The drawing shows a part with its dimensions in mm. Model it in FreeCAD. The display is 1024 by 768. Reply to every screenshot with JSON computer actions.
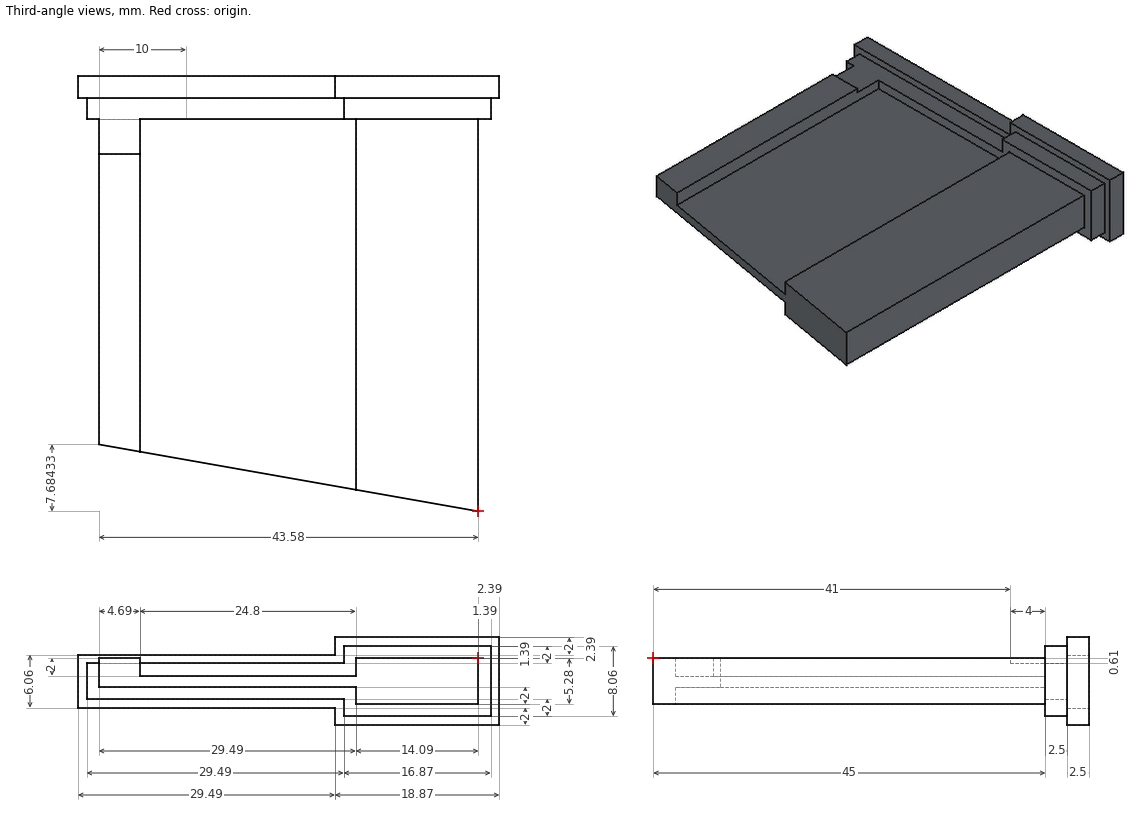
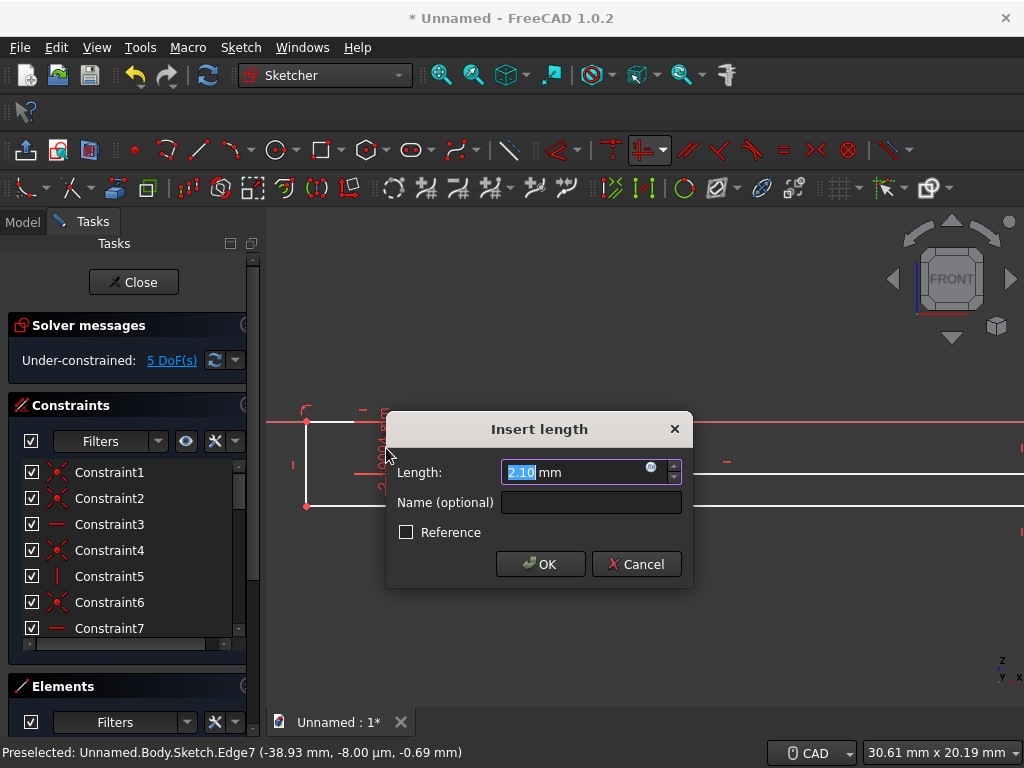
{"action": "type", "text": "2"}
{"action": "key", "text": "Return"}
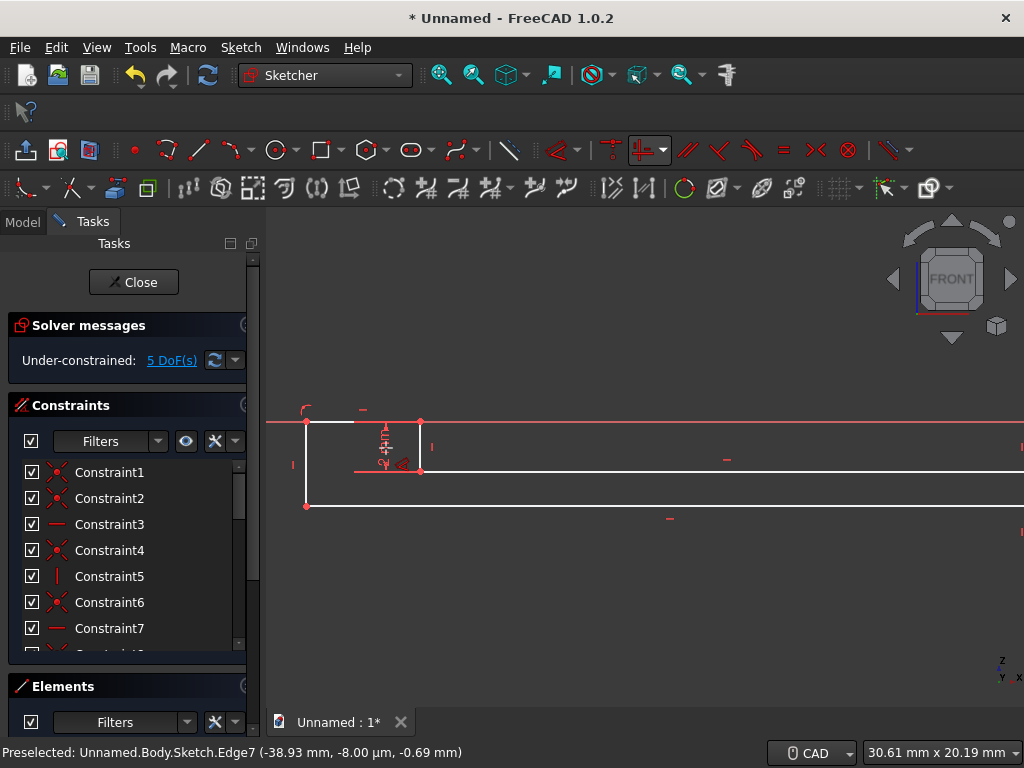
{"action": "scroll", "coordinate": [420, 439], "scroll_direction": "down", "scroll_amount": 5}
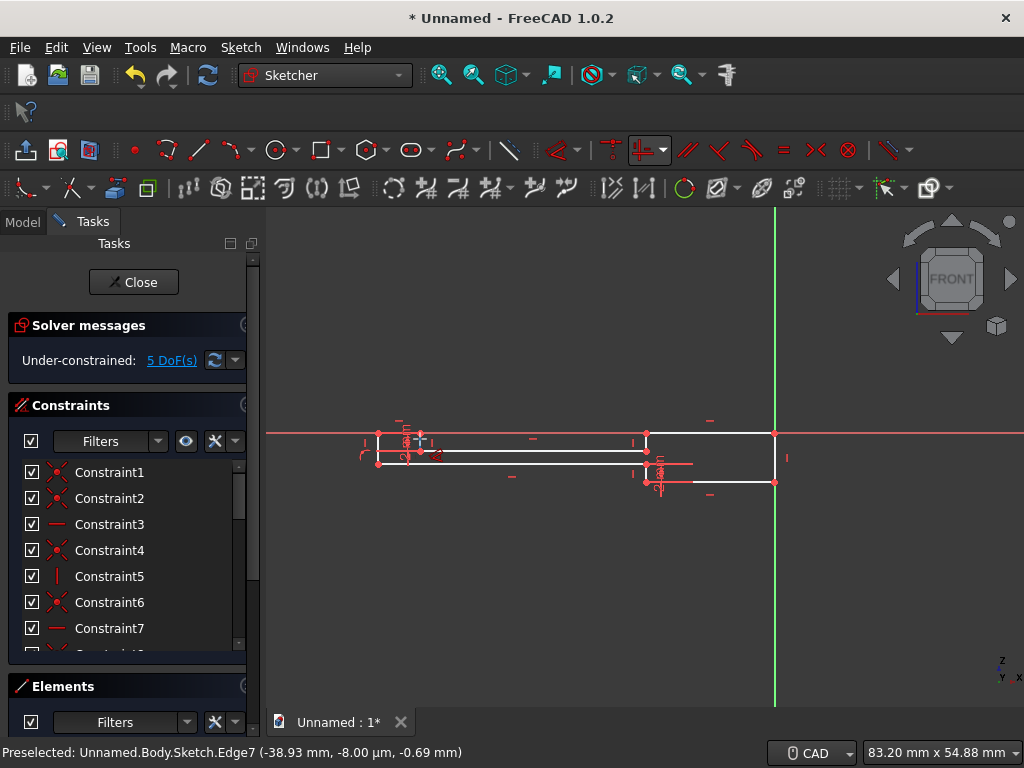
{"action": "left_click", "coordinate": [775, 448]}
{"action": "left_click", "coordinate": [809, 458]}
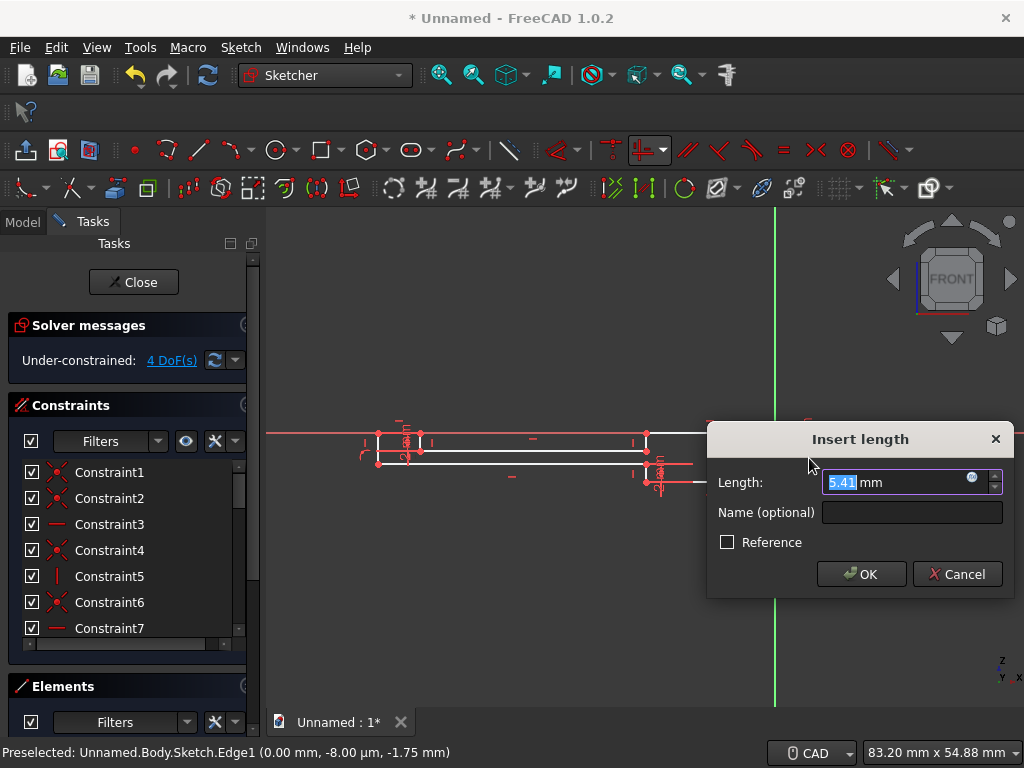
{"action": "type", "text": "5.28"}
{"action": "key", "text": "Return"}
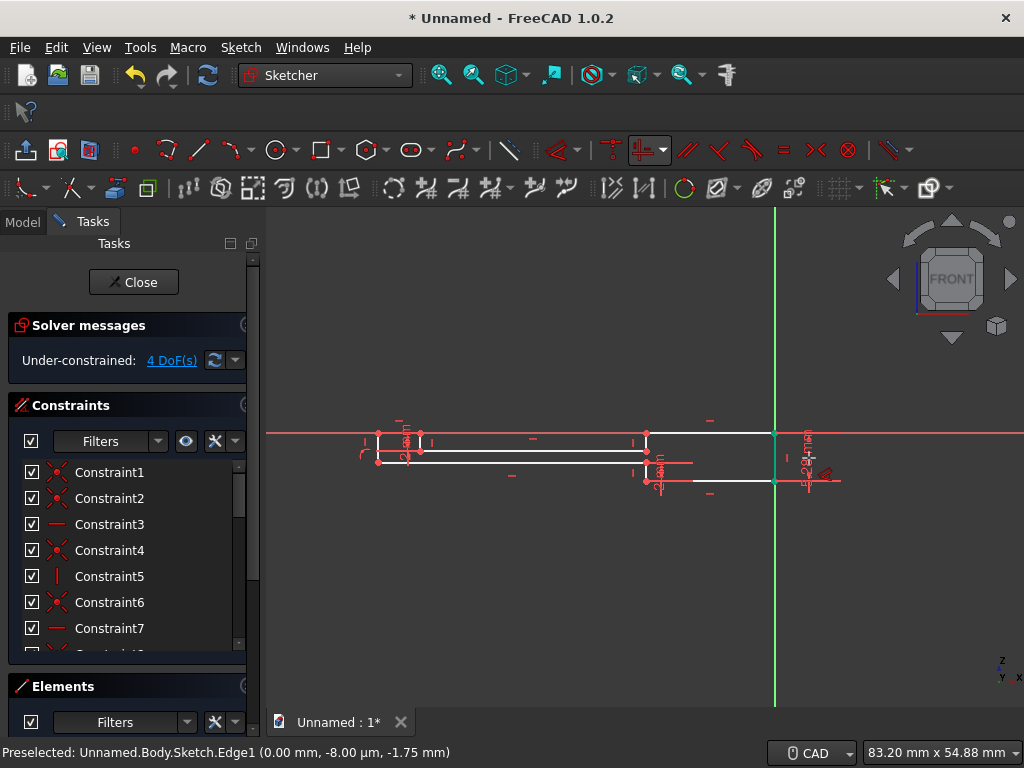
{"action": "left_click", "coordinate": [391, 433]}
{"action": "left_click", "coordinate": [399, 399]}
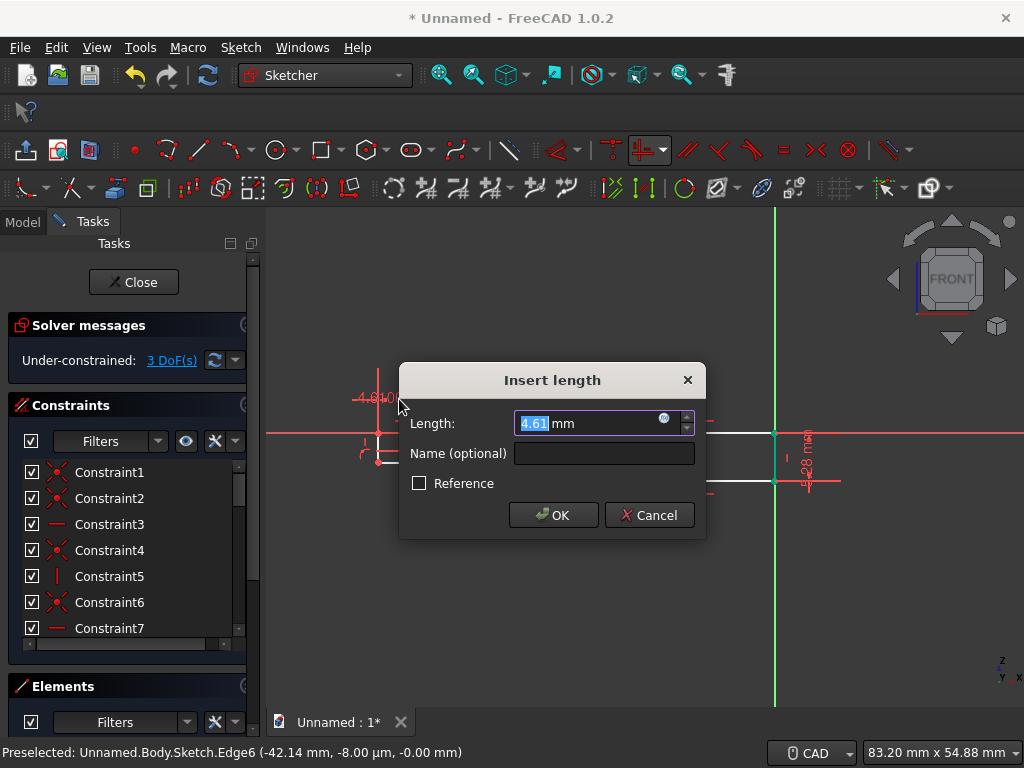
{"action": "type", "text": "4.69"}
{"action": "key", "text": "Return"}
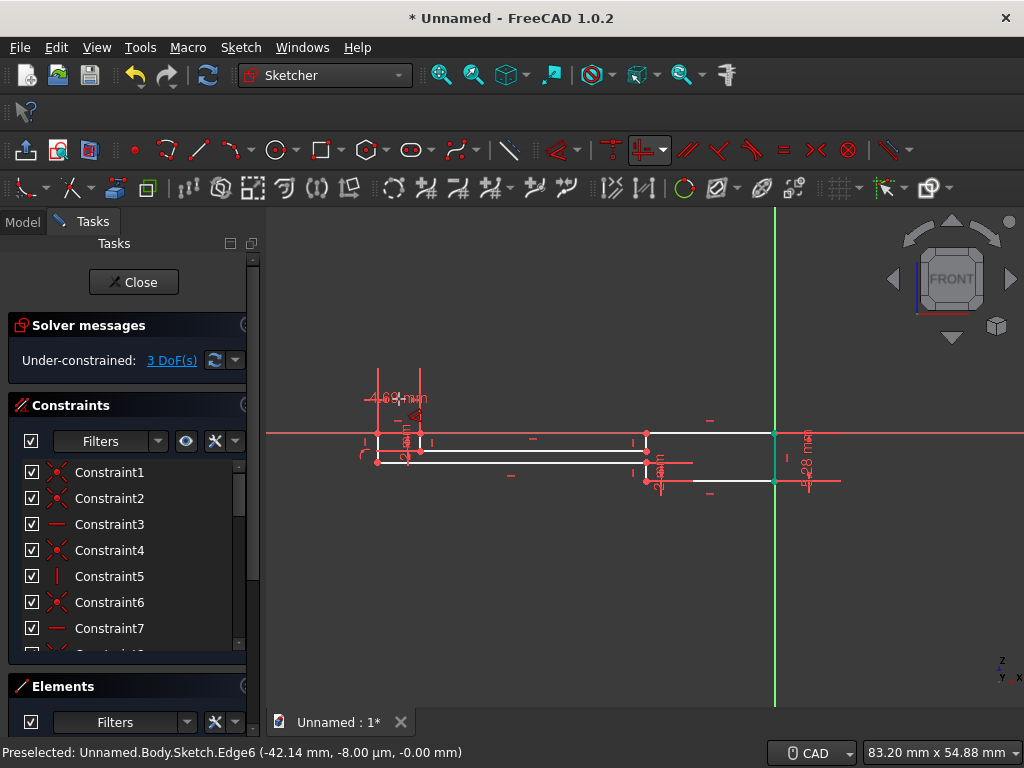
{"action": "left_click", "coordinate": [488, 451]}
{"action": "left_click", "coordinate": [533, 417]}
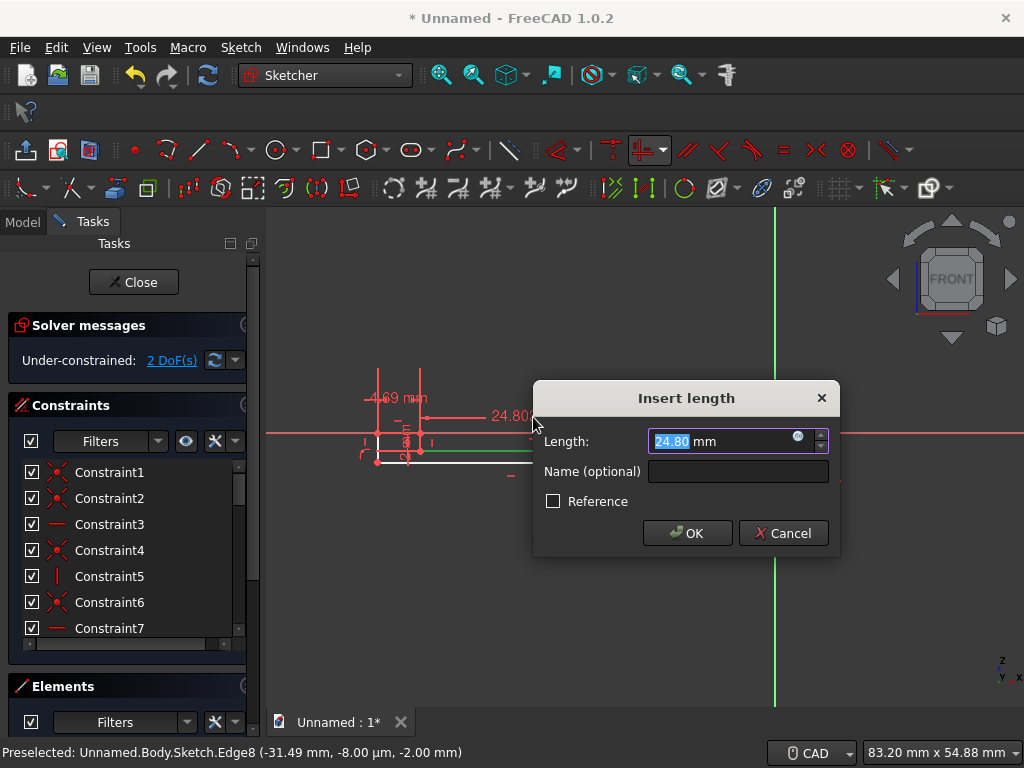
{"action": "type", "text": "24.8"}
{"action": "key", "text": "Return"}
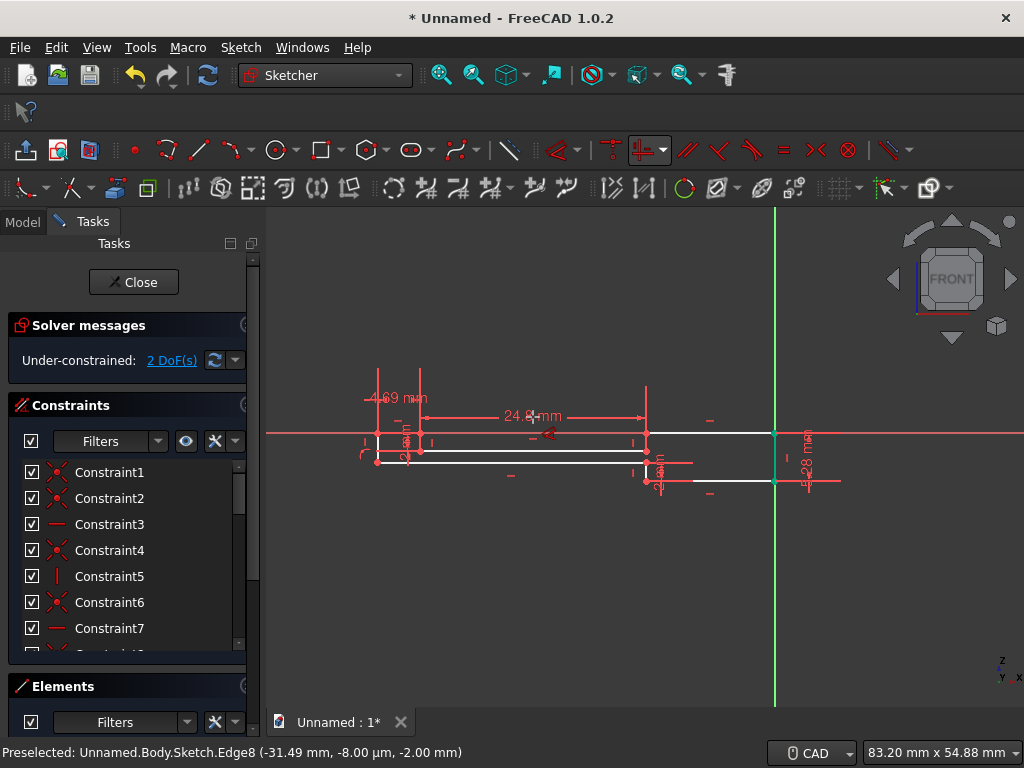
{"action": "left_click", "coordinate": [736, 481]}
{"action": "left_click", "coordinate": [711, 515]}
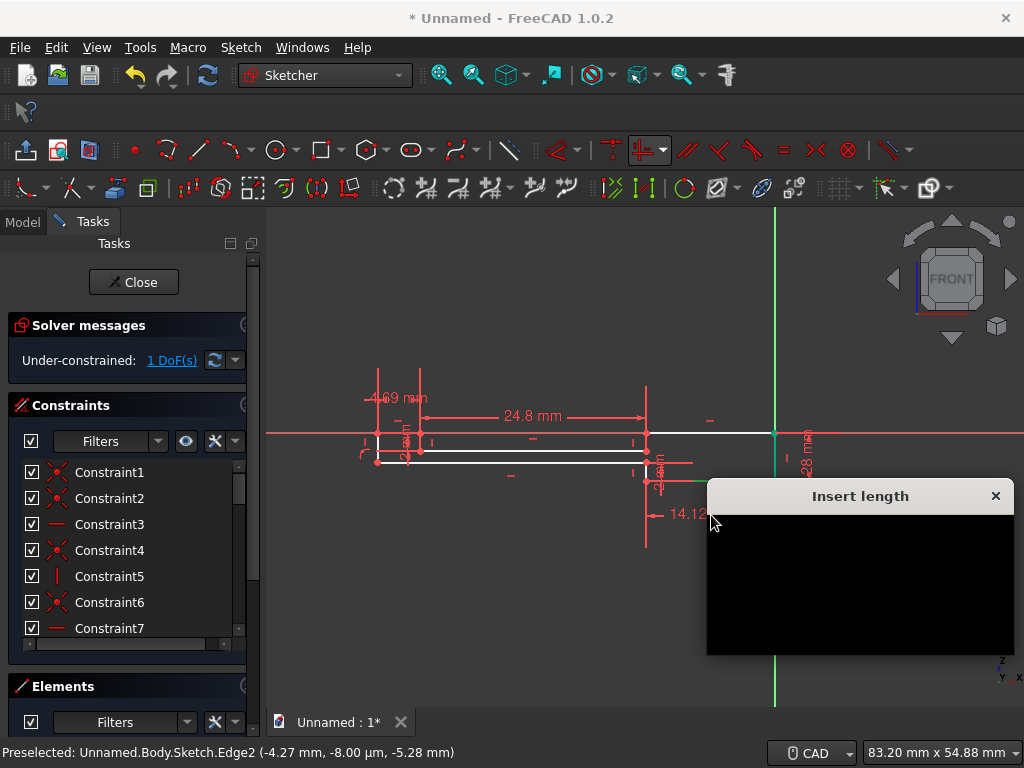
{"action": "type", "text": "14.09"}
{"action": "key", "text": "Return"}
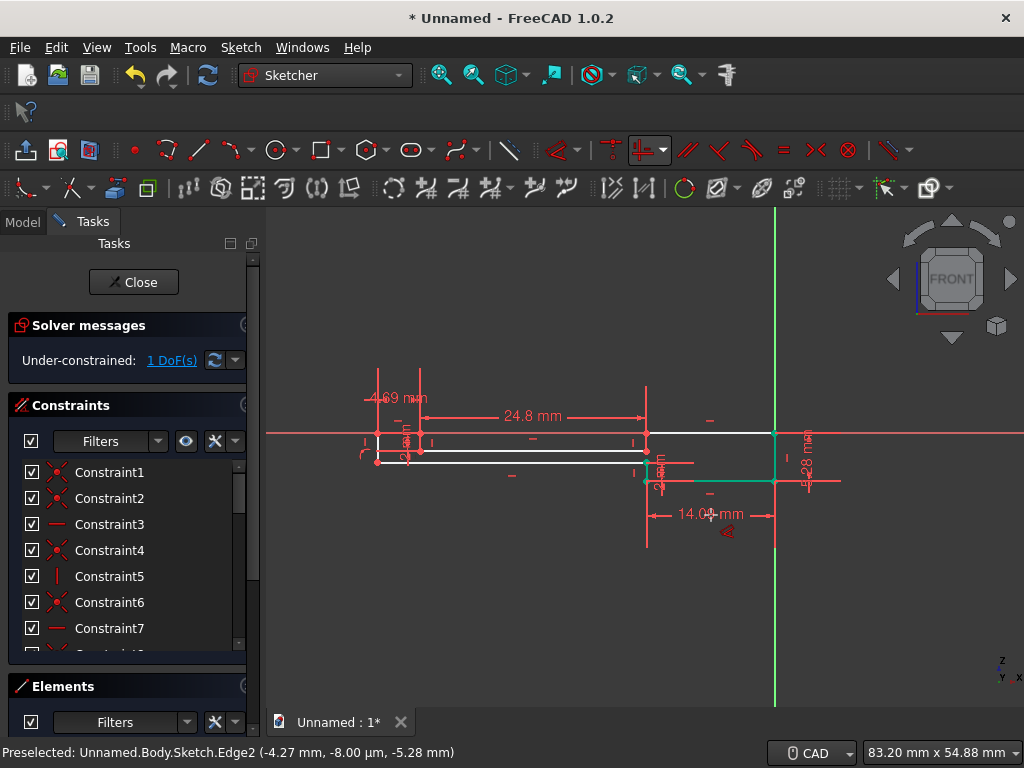
{"action": "left_click", "coordinate": [566, 463]}
{"action": "left_click", "coordinate": [512, 497]}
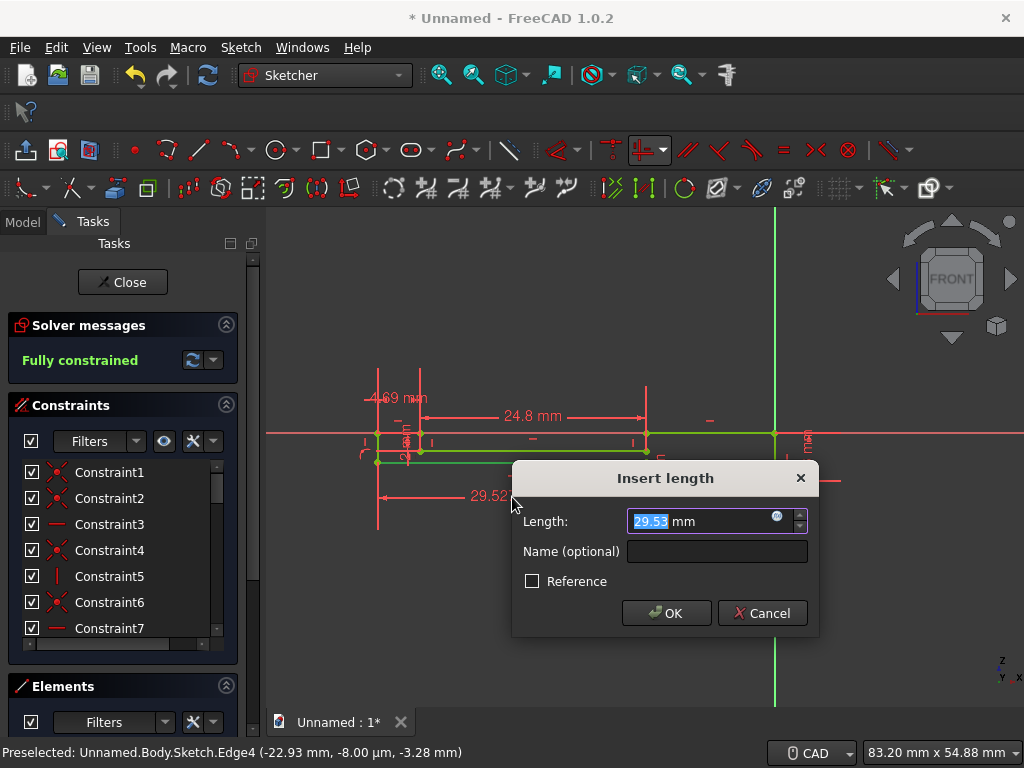
{"action": "type", "text": "29.49"}
{"action": "key", "text": "Return"}
{"action": "key", "text": "Escape"}